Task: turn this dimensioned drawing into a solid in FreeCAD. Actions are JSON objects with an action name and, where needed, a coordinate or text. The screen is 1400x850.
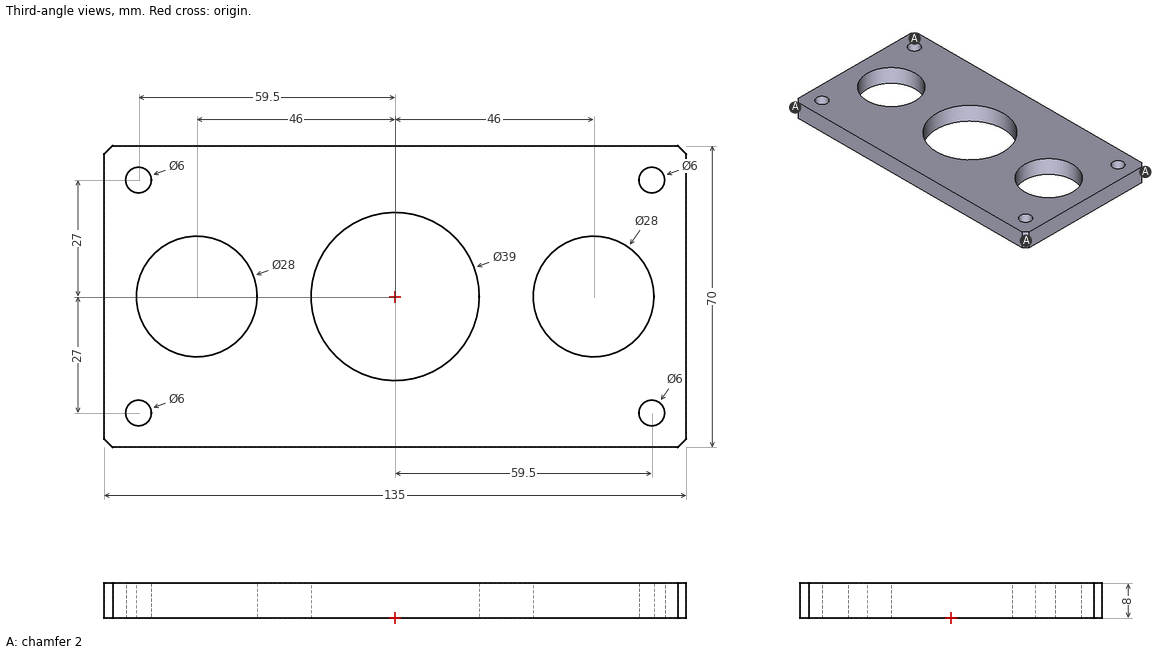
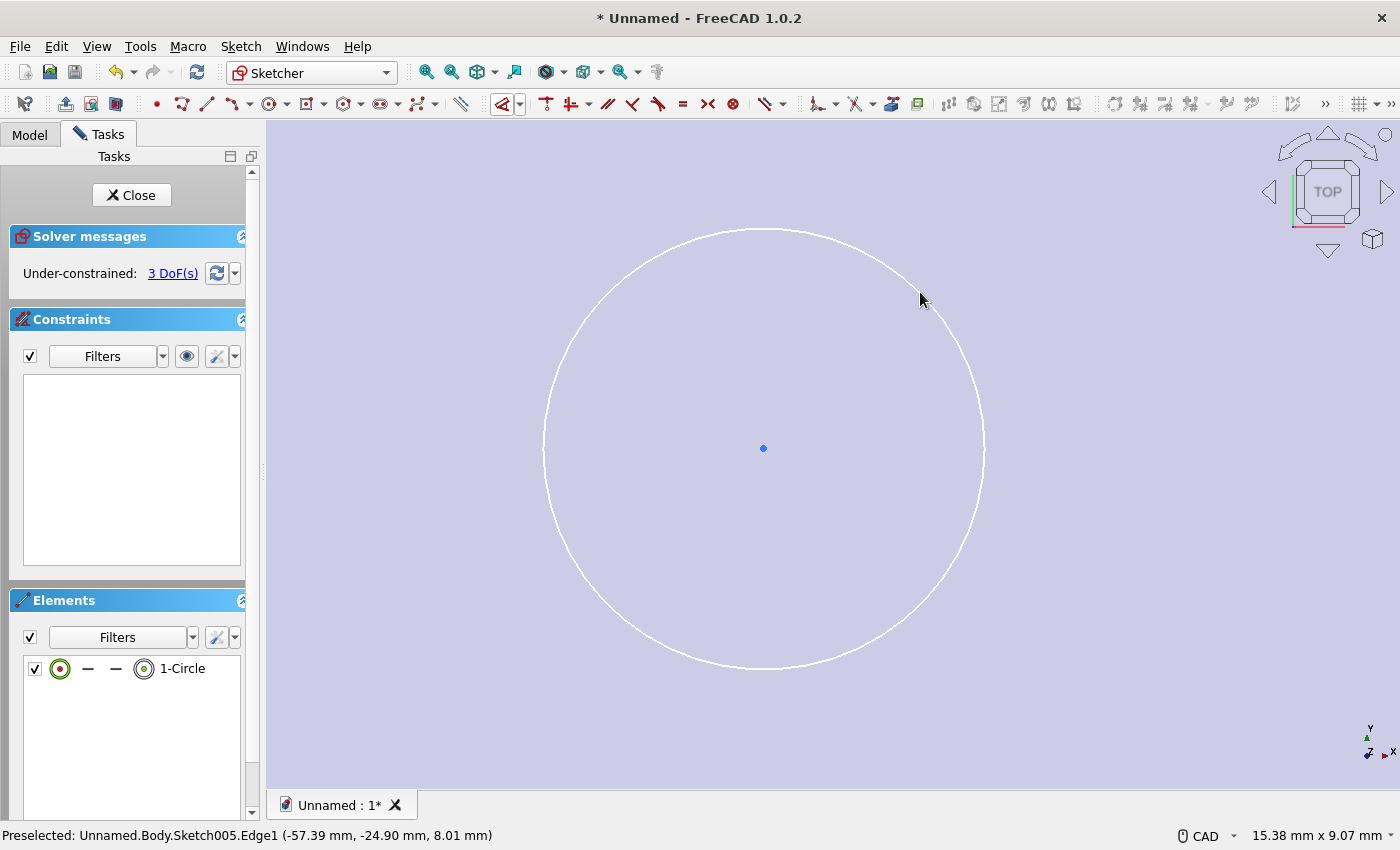
{"action": "left_click", "coordinate": [920, 293]}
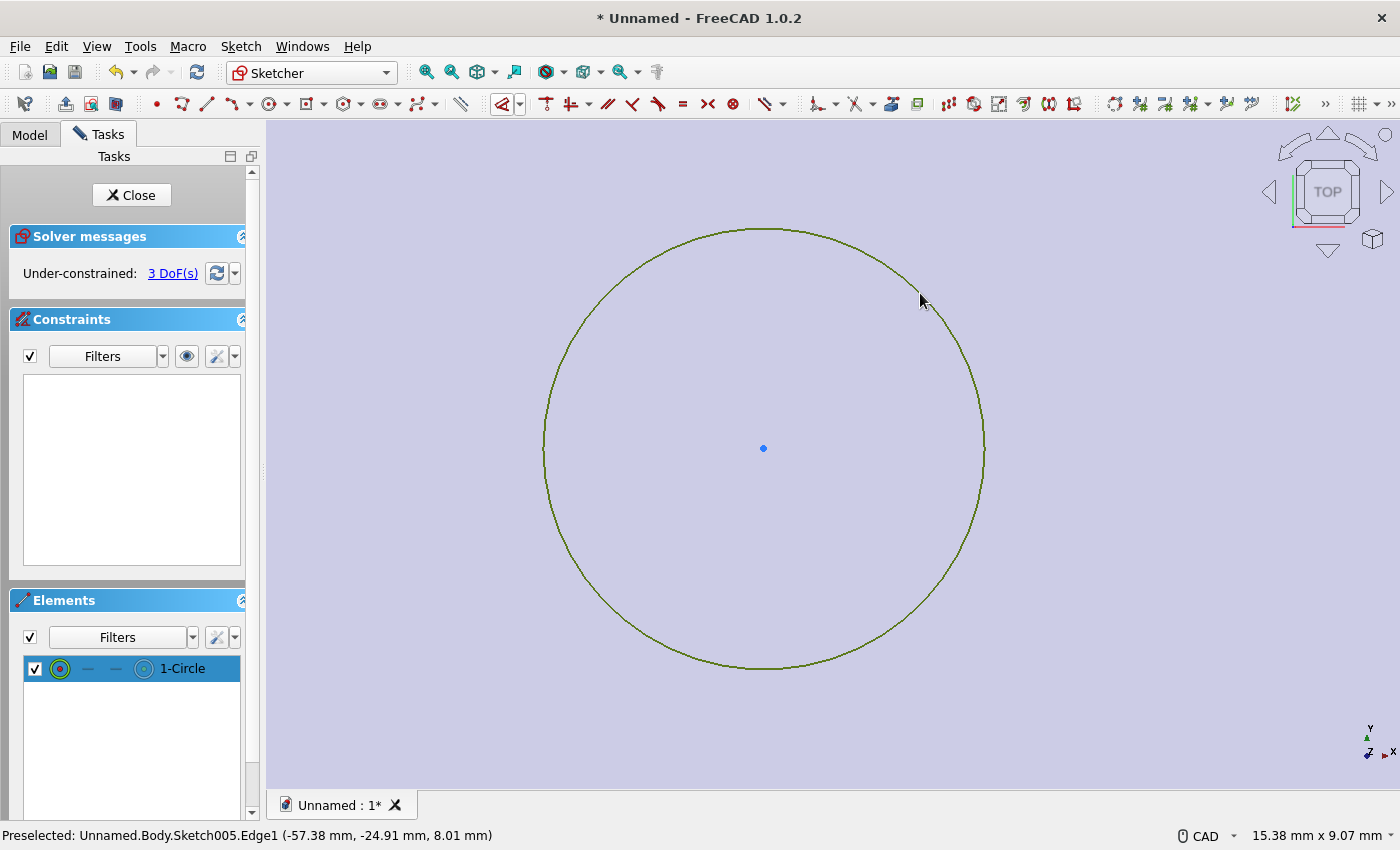
{"action": "key", "text": "k o"}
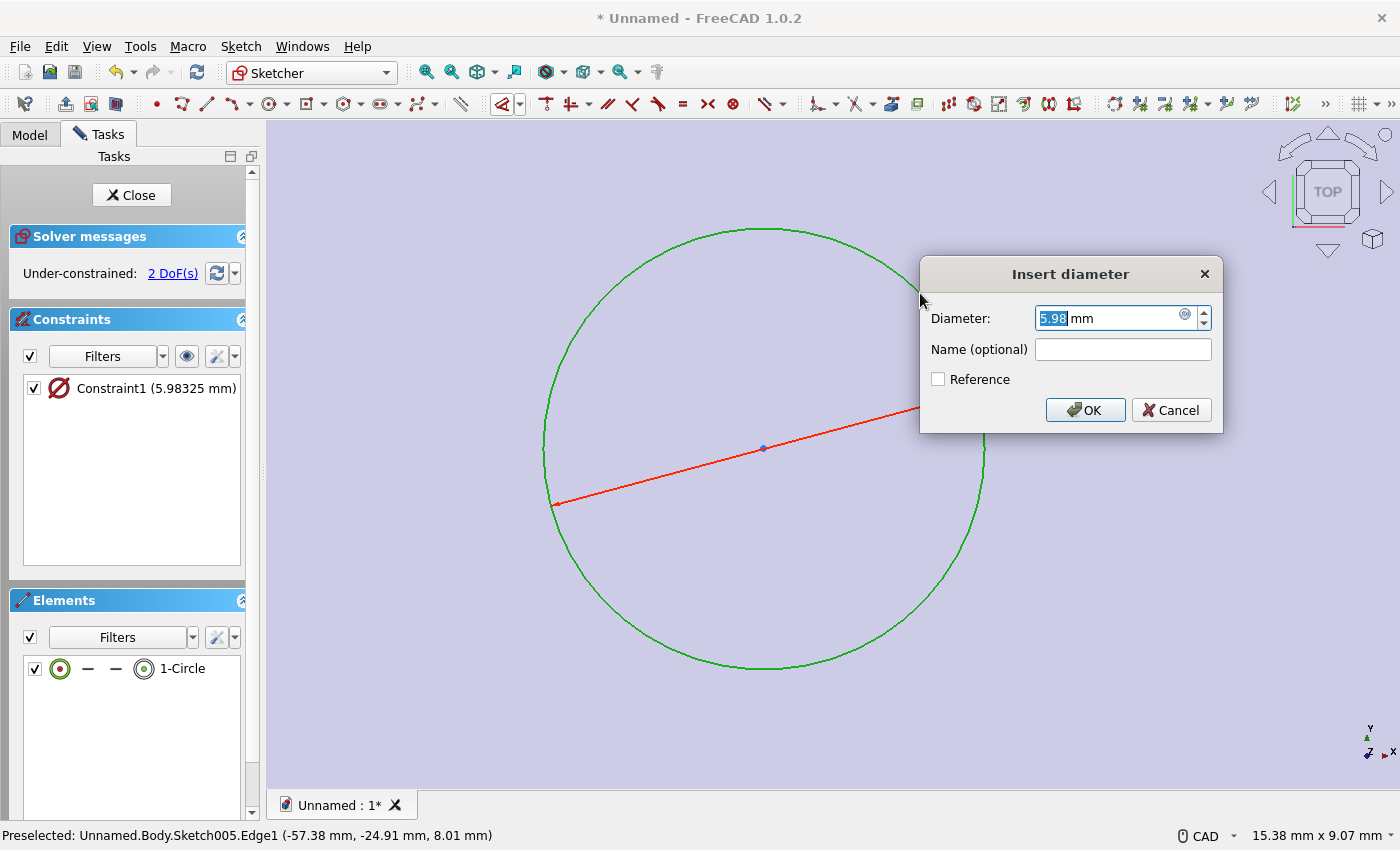
{"action": "type", "text": "6"}
{"action": "key", "text": "Return"}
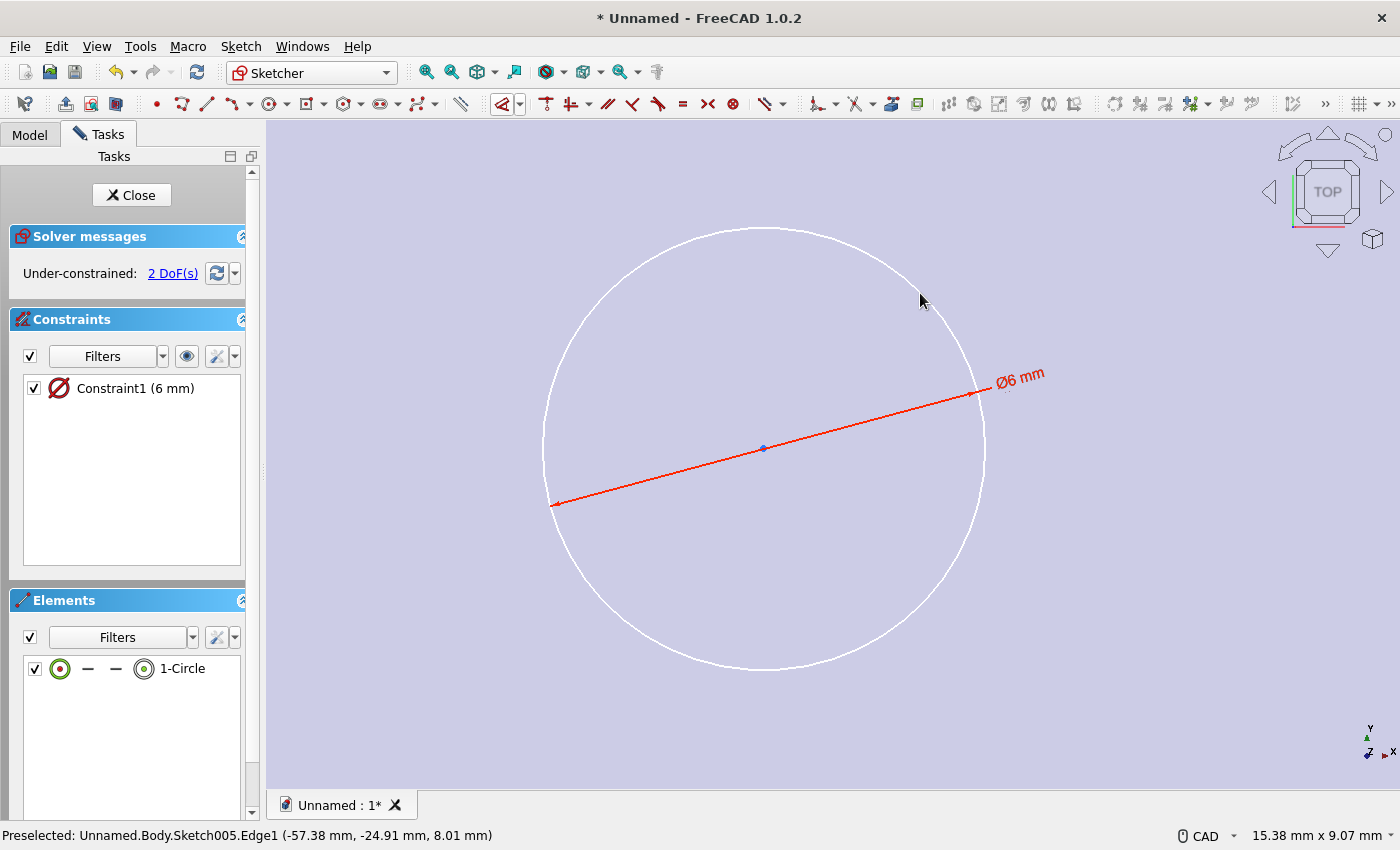
{"action": "left_click", "coordinate": [764, 449]}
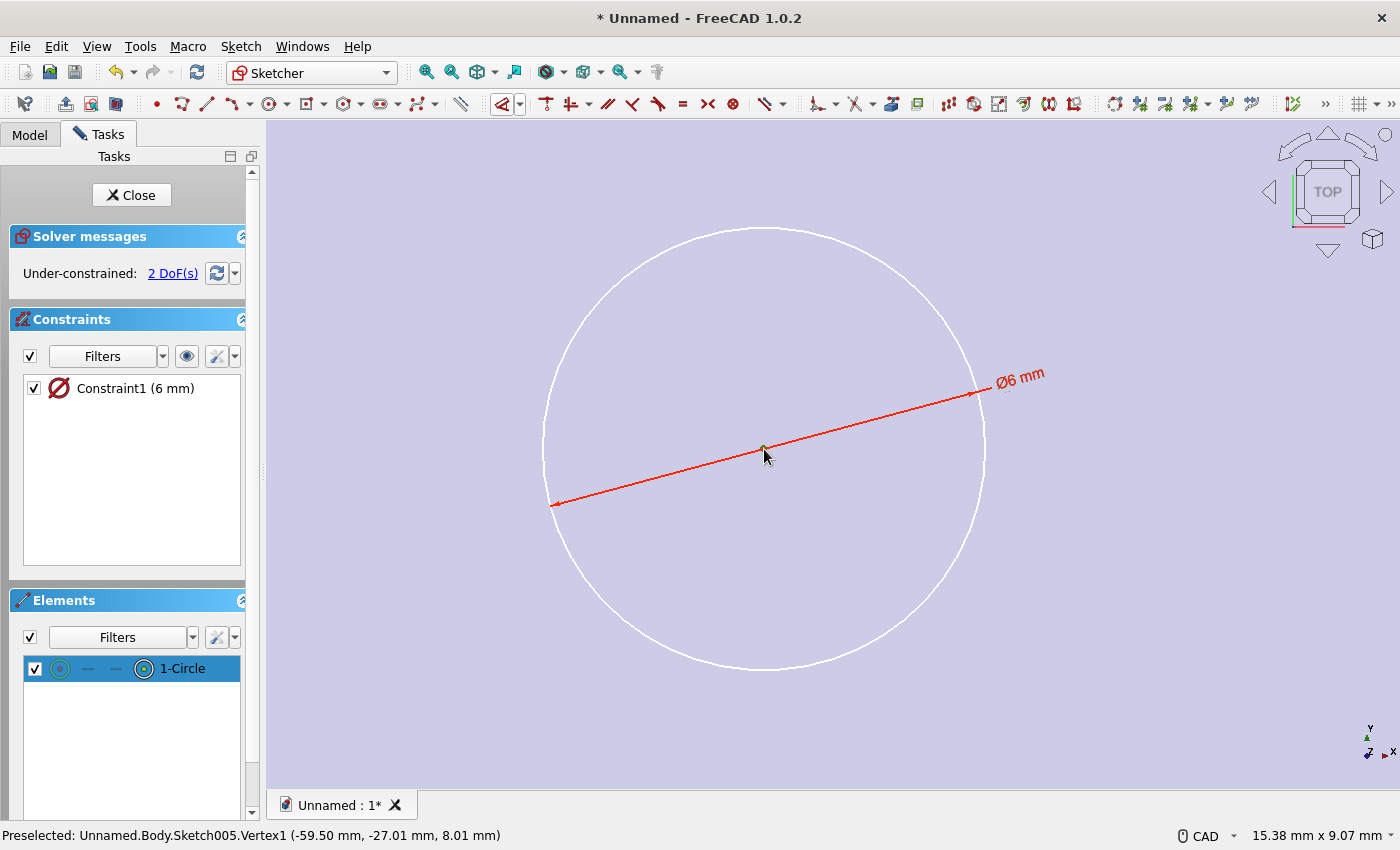
{"action": "key", "text": "i"}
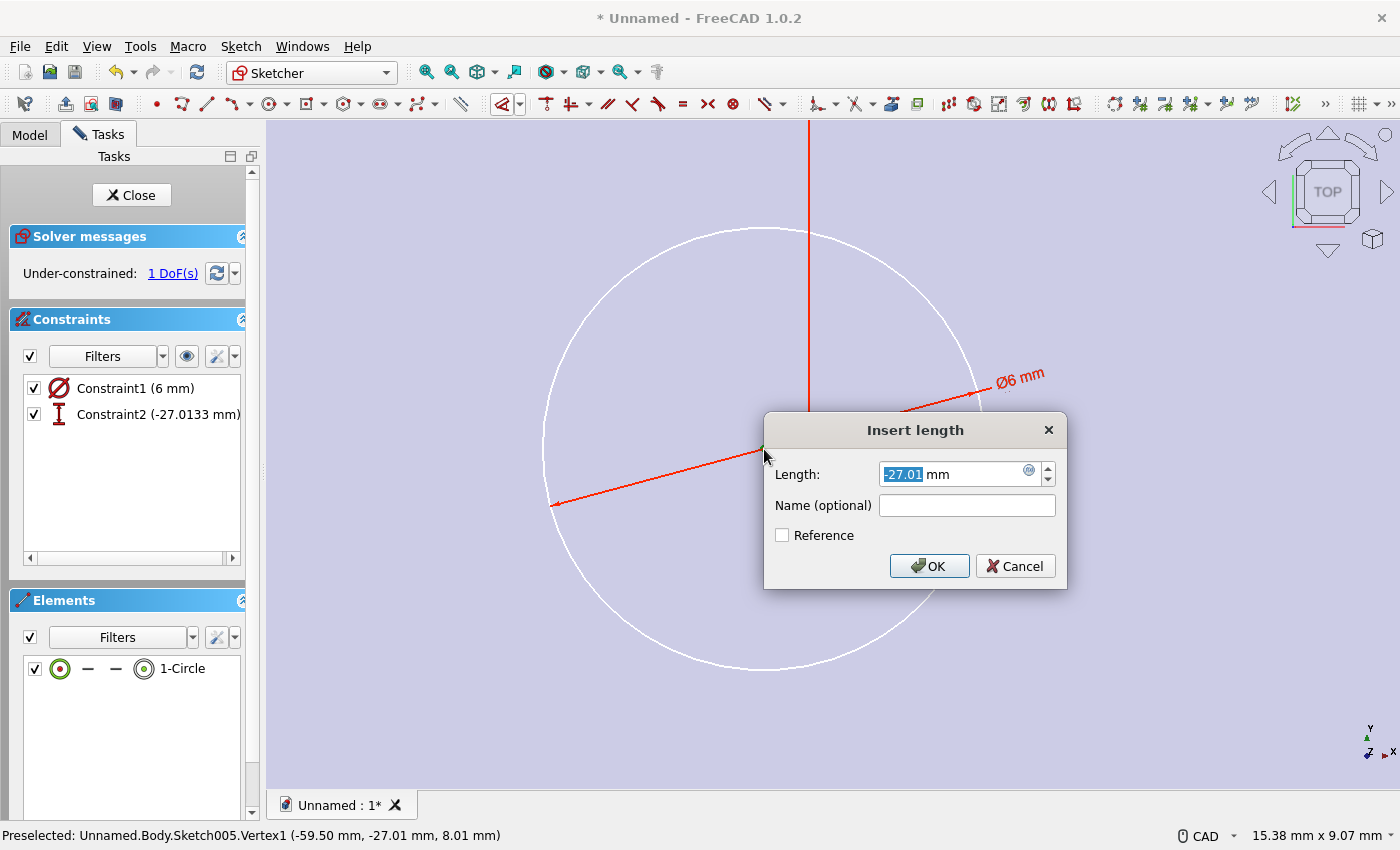
{"action": "type", "text": "-27"}
{"action": "key", "text": "Return"}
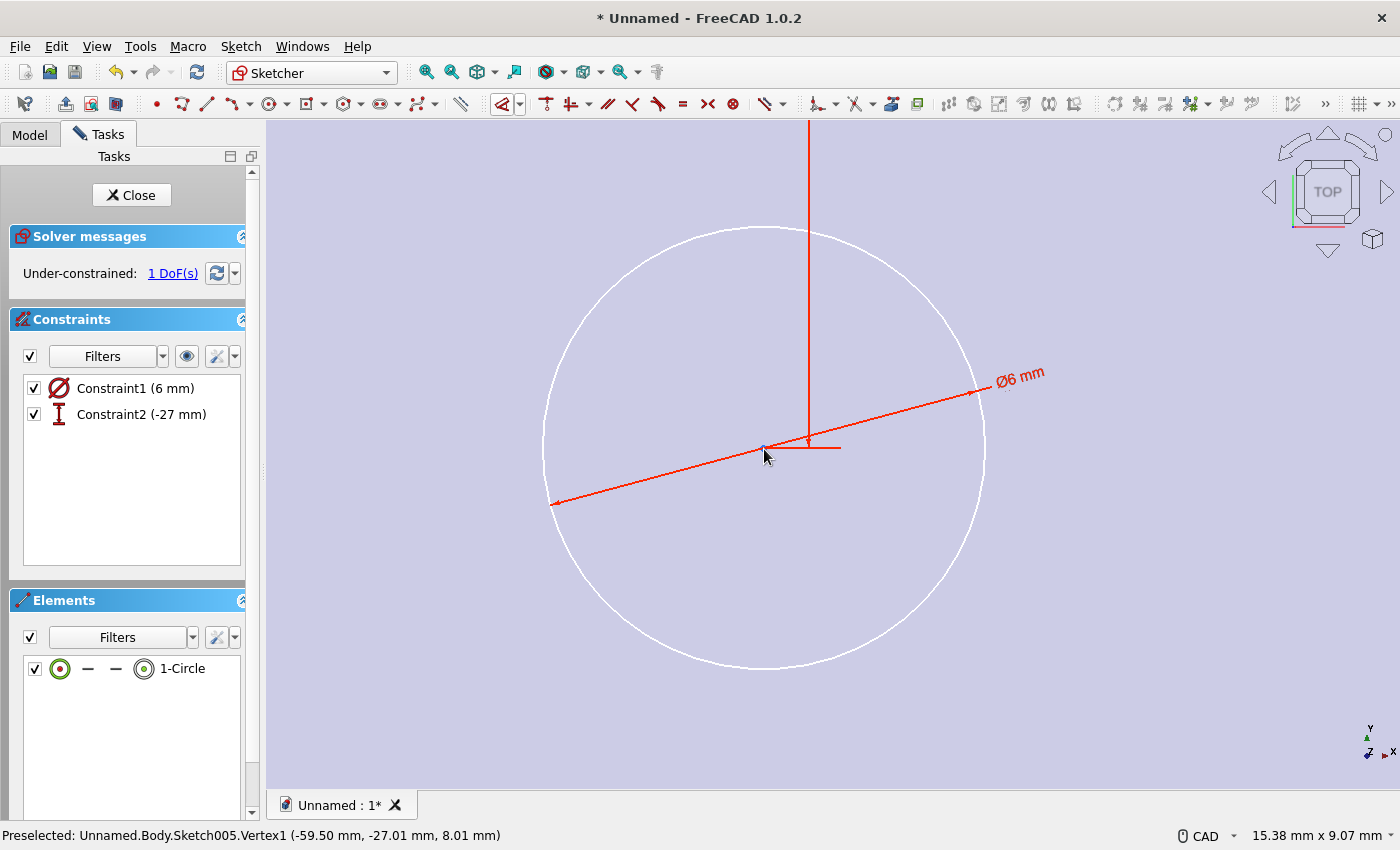
{"action": "left_click", "coordinate": [764, 448]}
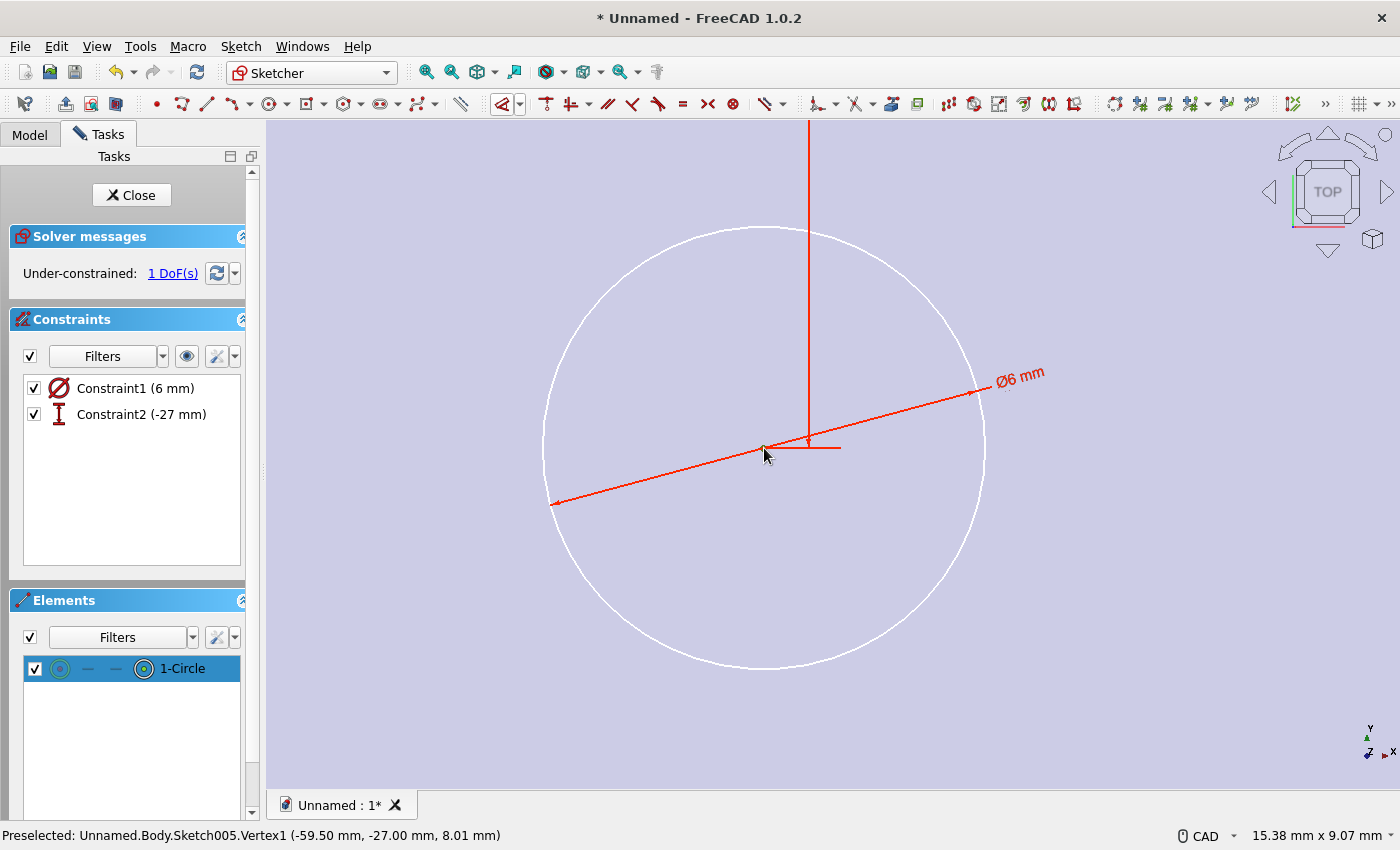
{"action": "left_click", "coordinate": [520, 104]}